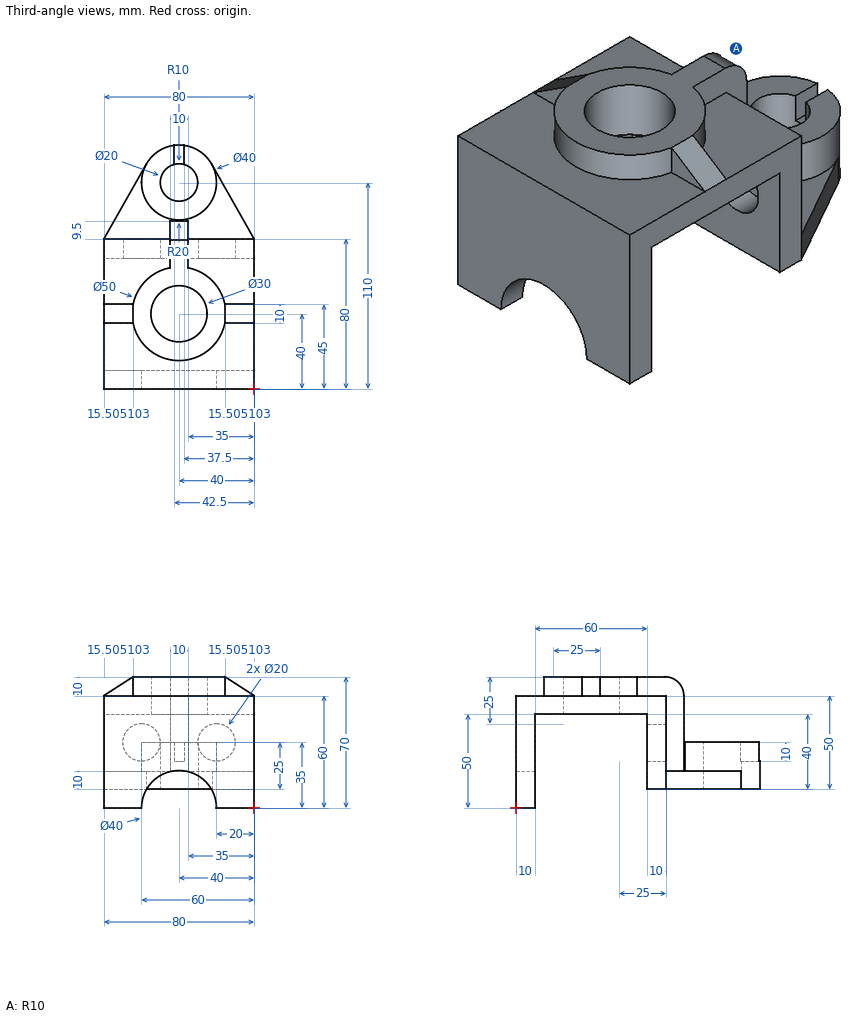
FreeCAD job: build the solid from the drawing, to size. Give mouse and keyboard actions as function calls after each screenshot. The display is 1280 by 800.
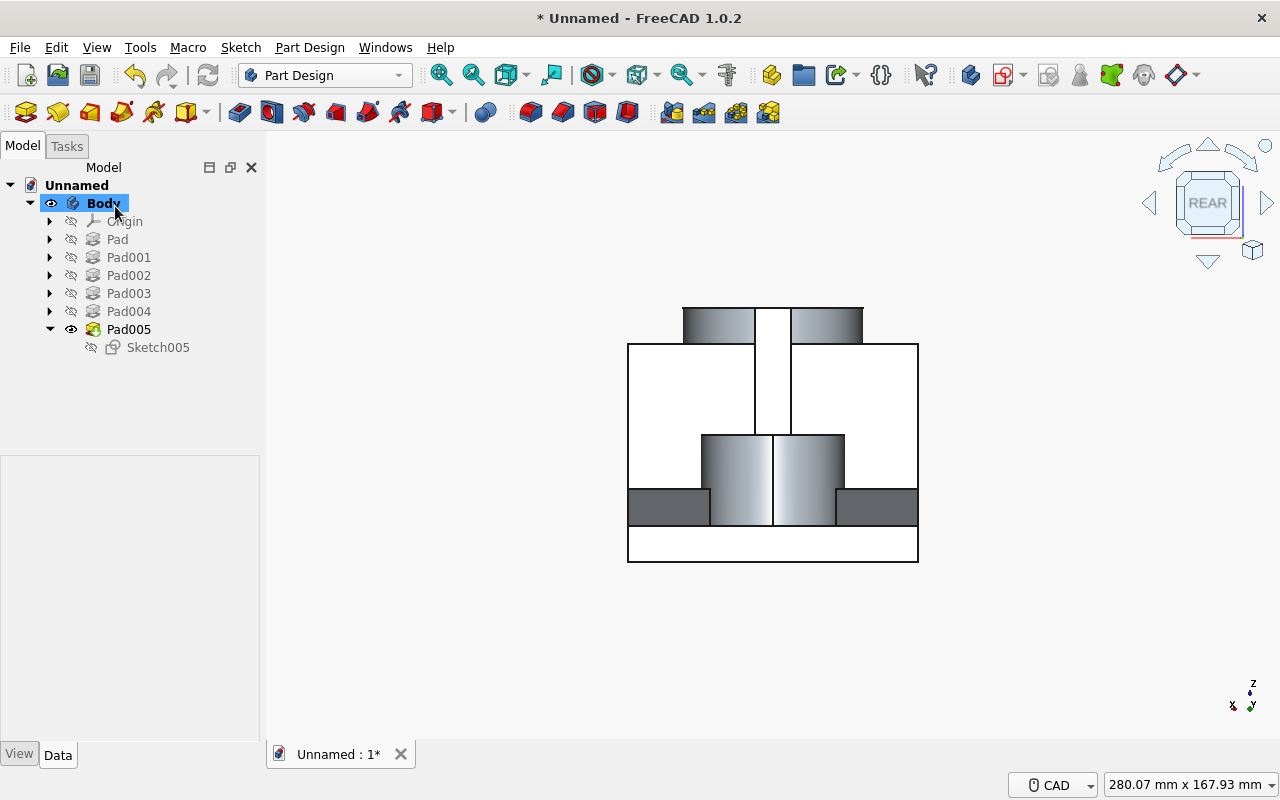
click(442, 76)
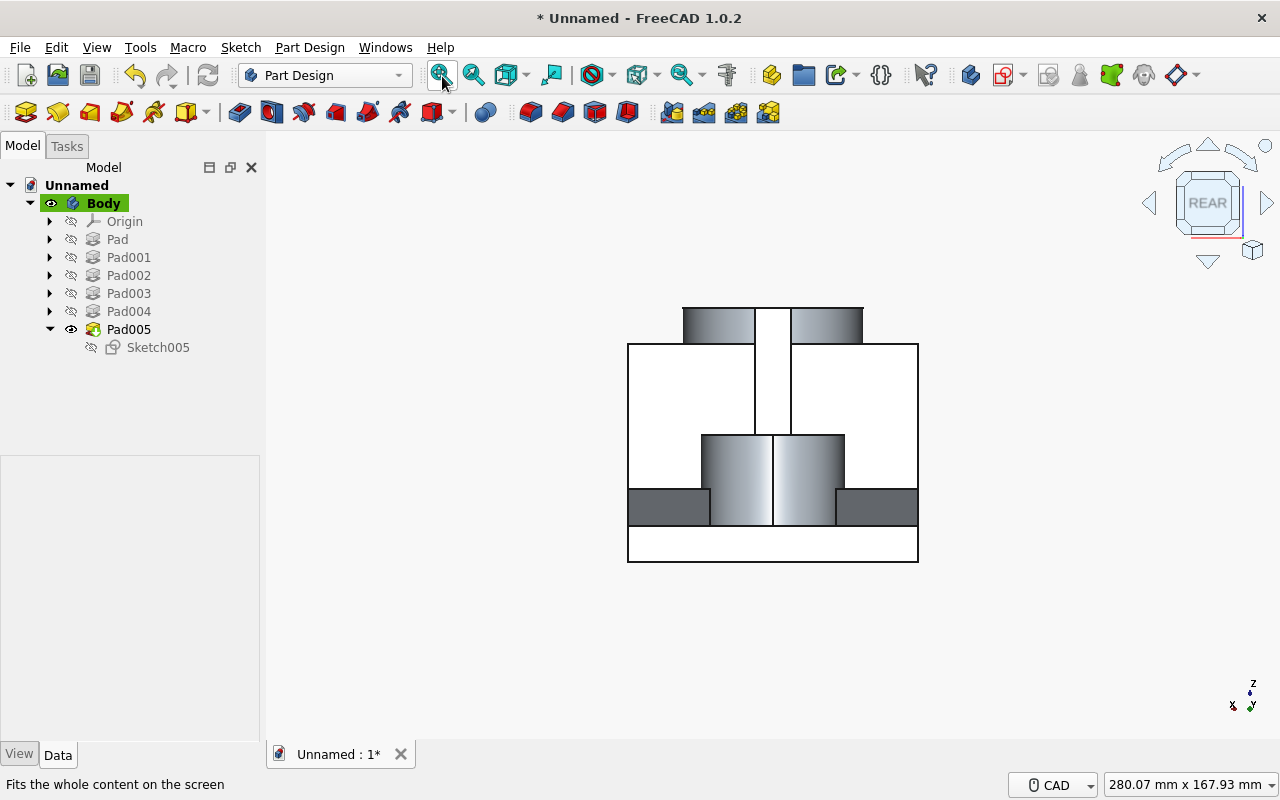
click(773, 307)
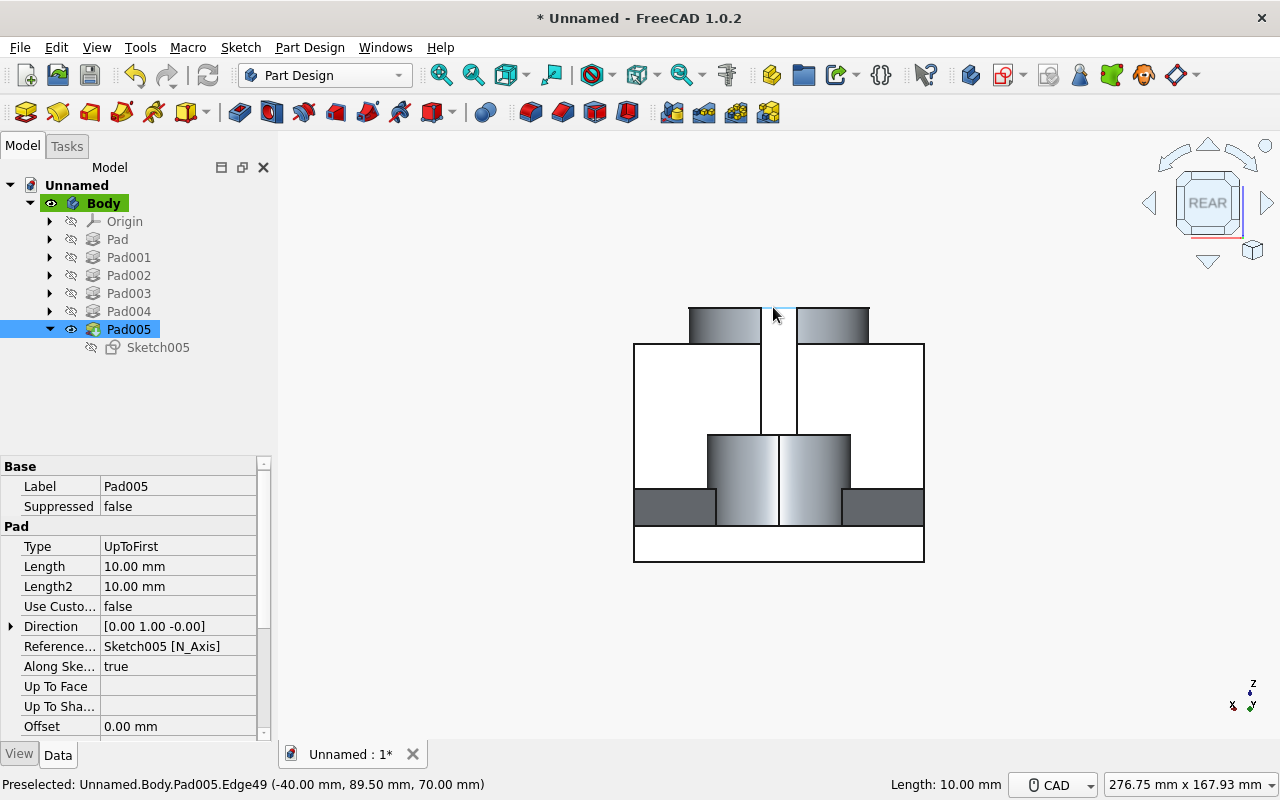
click(532, 112)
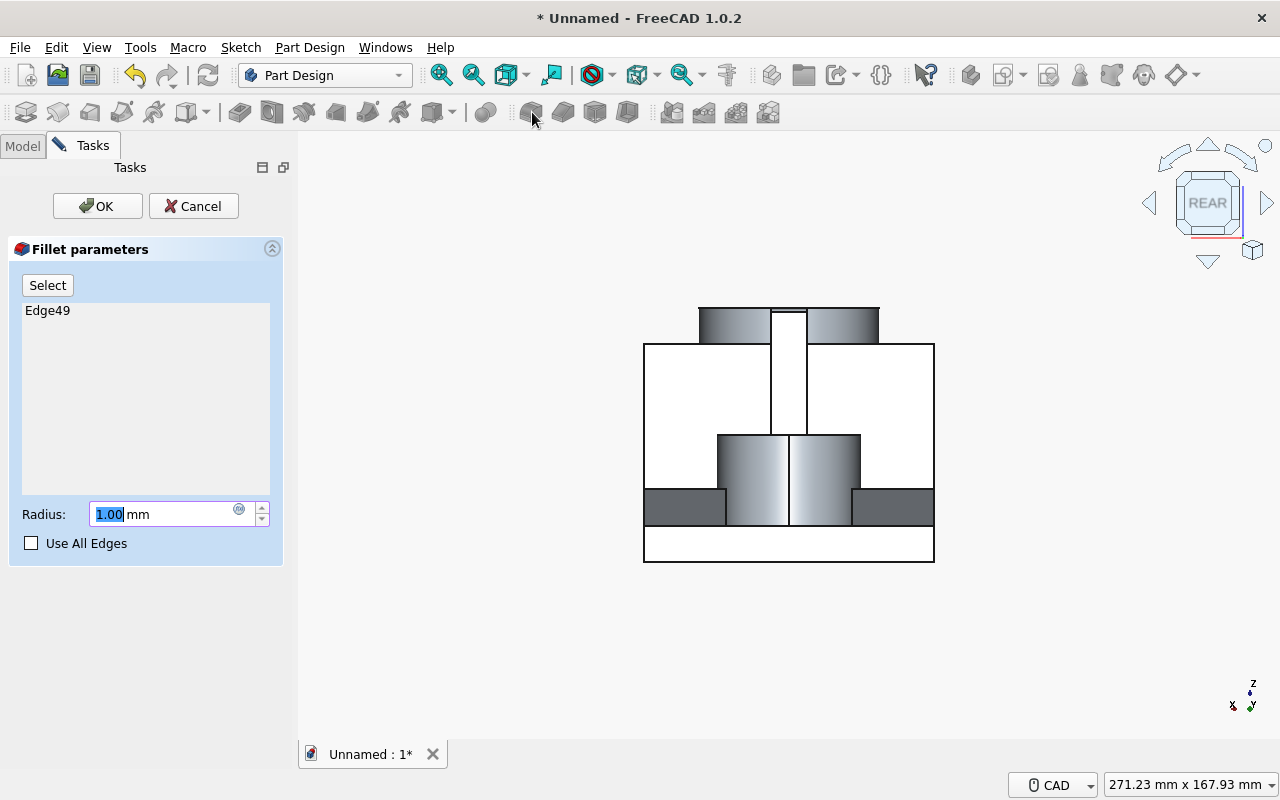
text(10)
key(Tab)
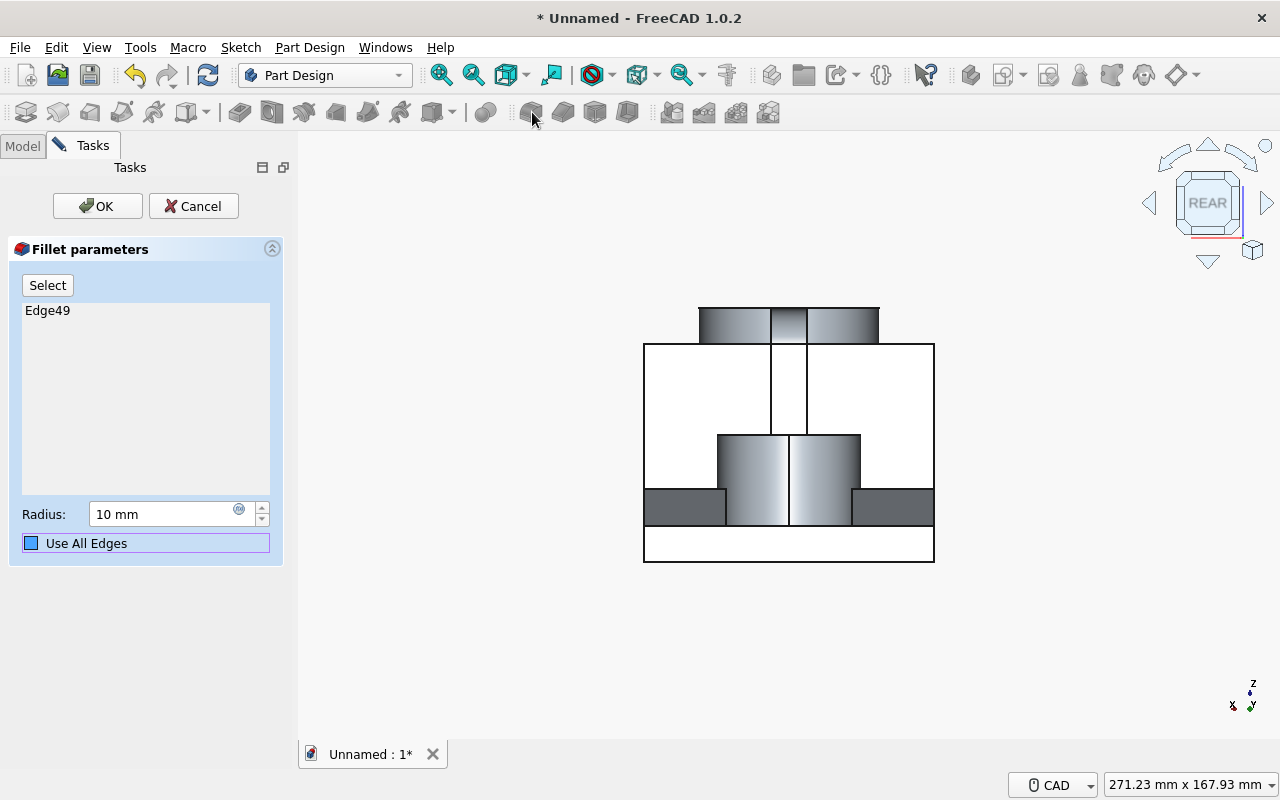
click(98, 206)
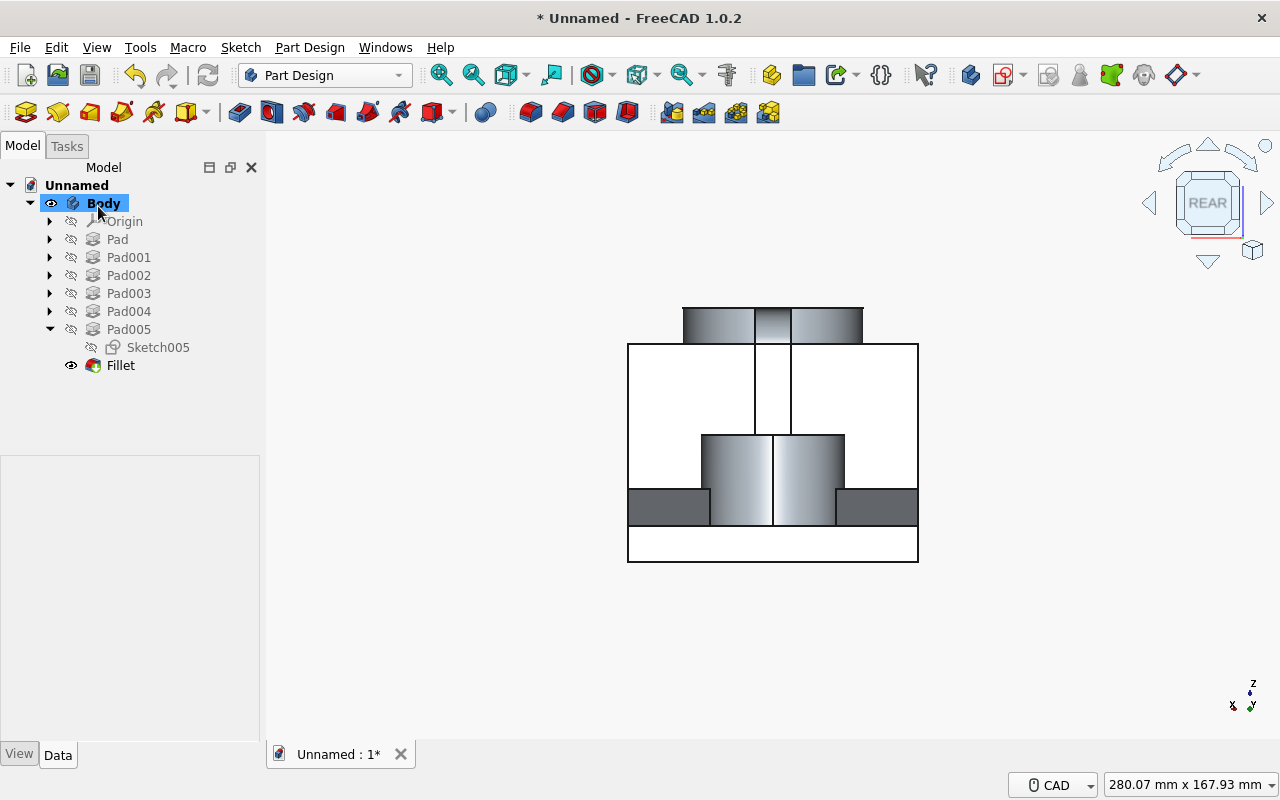
click(442, 76)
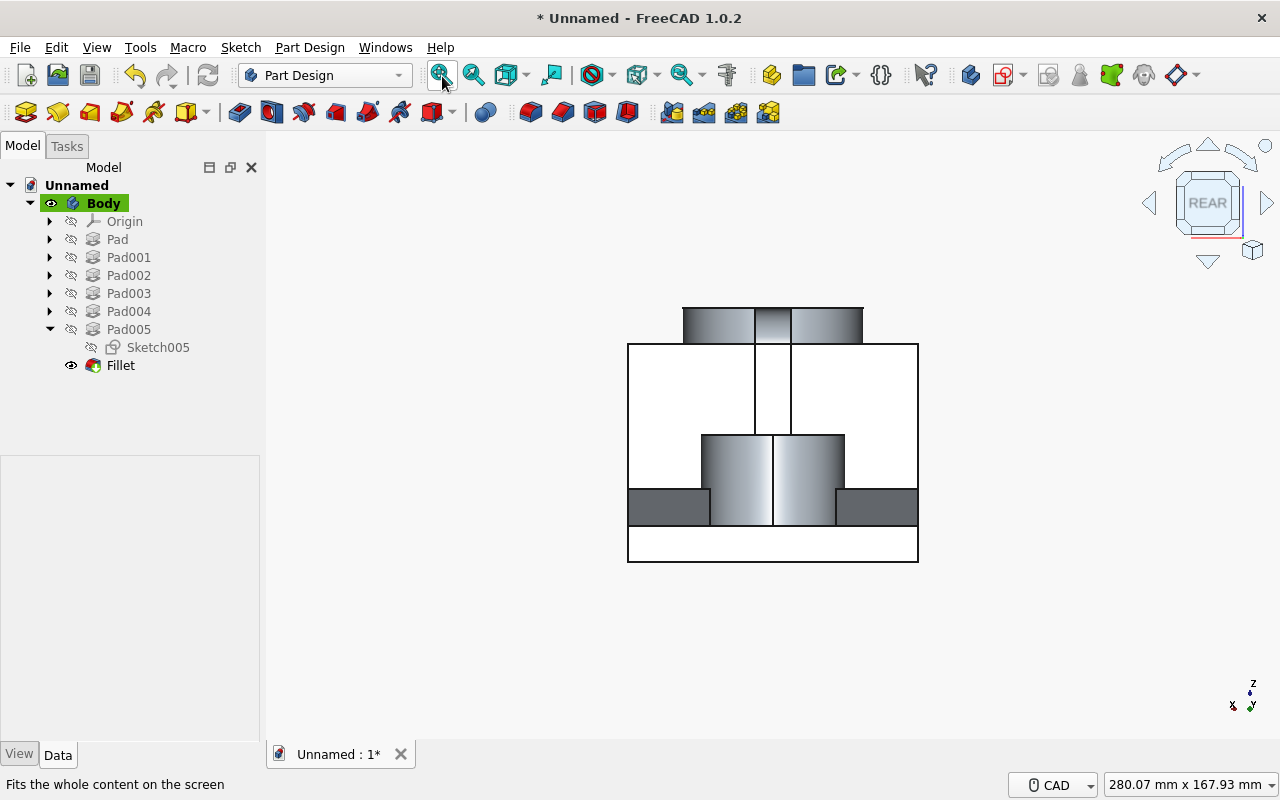
key(0)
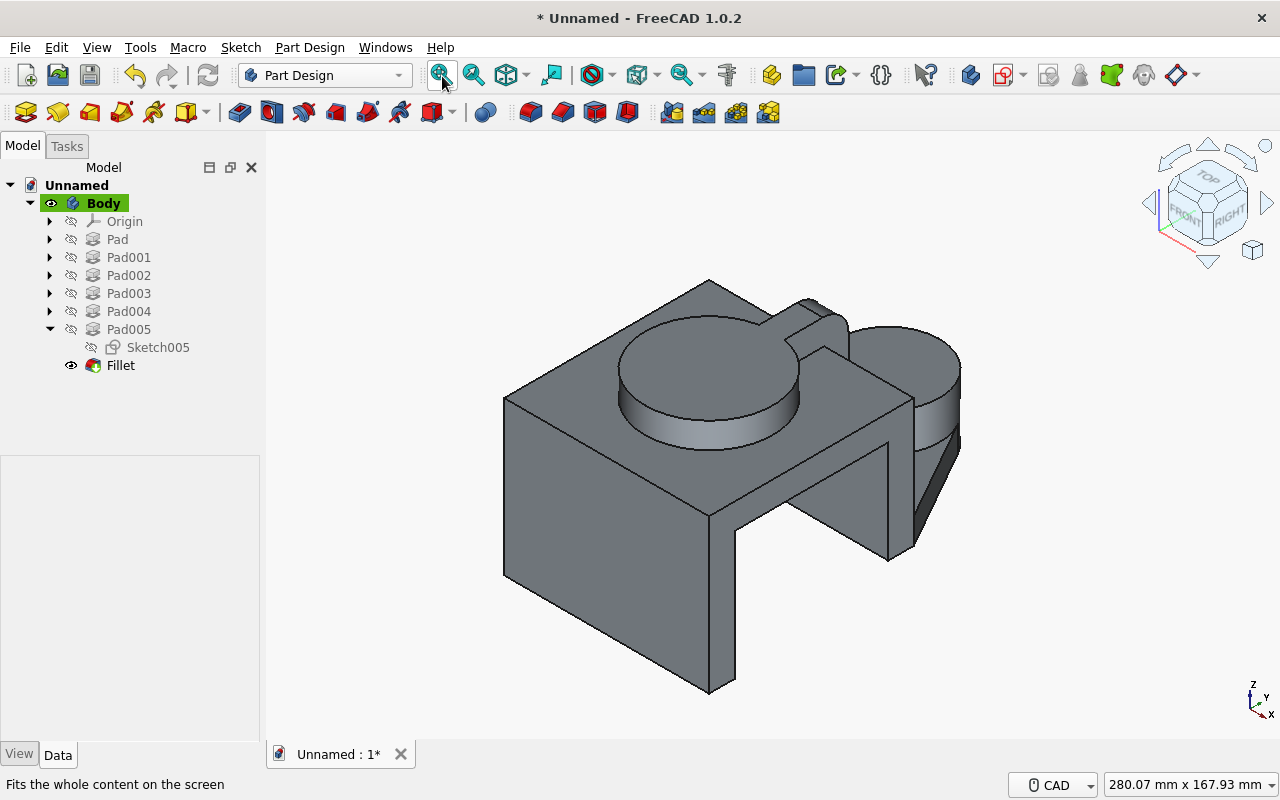
click(704, 370)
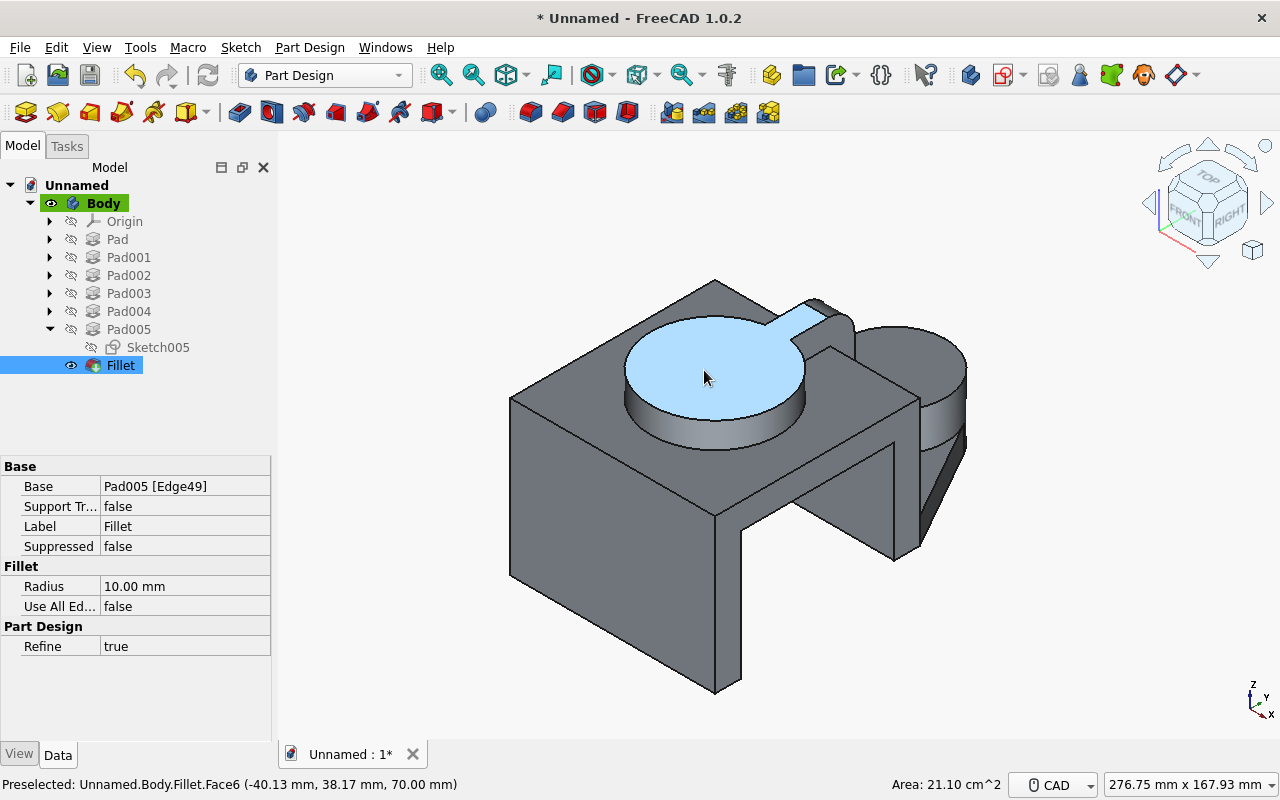
click(1004, 76)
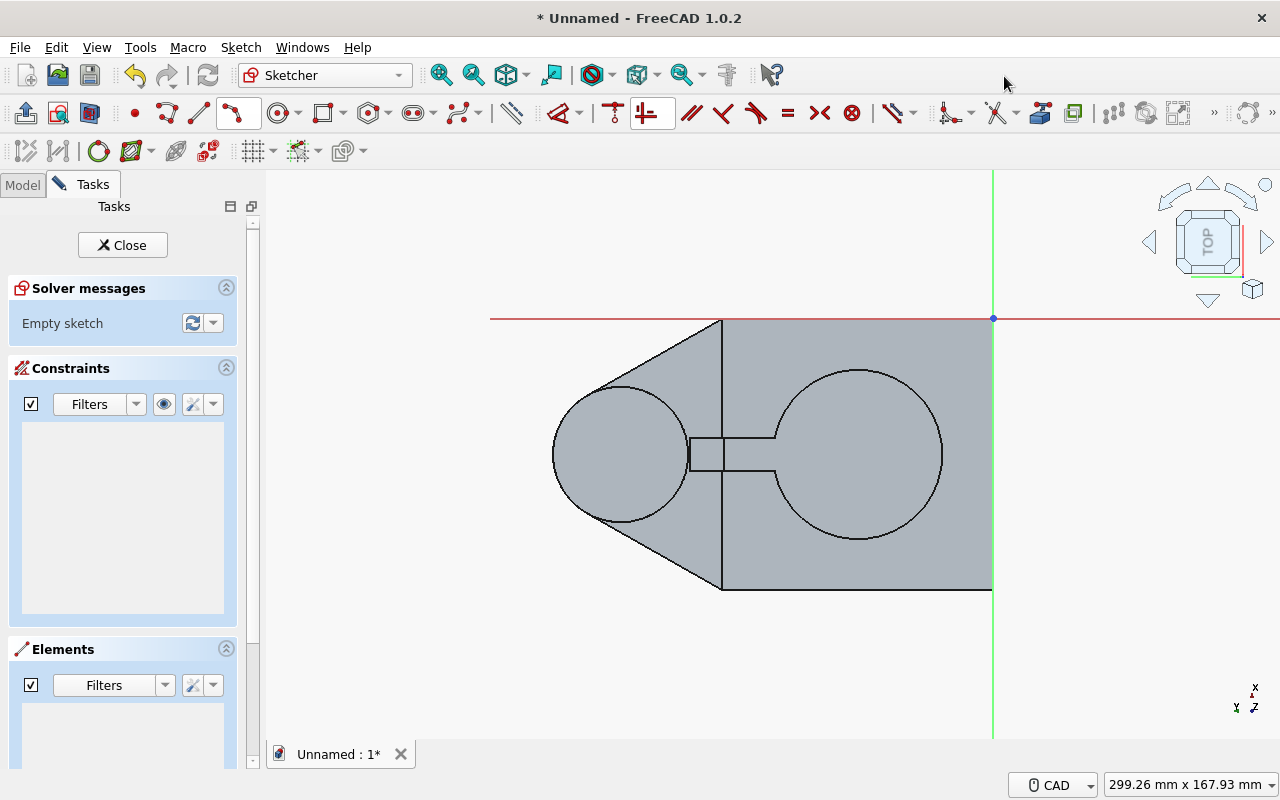
scroll(882, 328, up, 10)